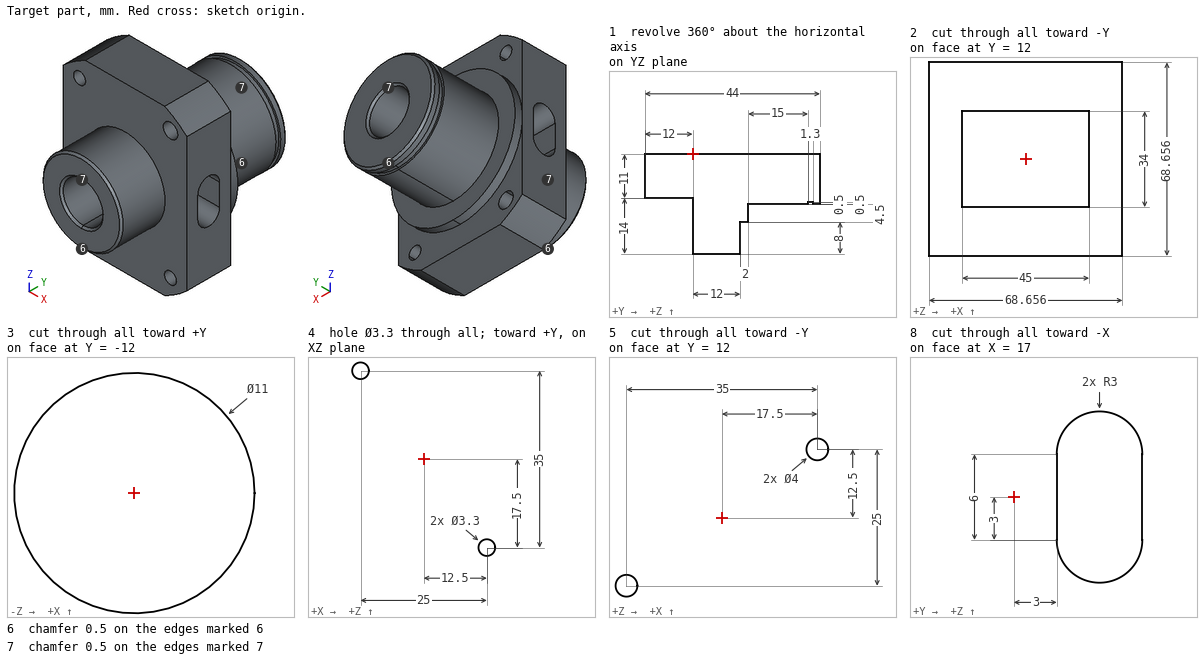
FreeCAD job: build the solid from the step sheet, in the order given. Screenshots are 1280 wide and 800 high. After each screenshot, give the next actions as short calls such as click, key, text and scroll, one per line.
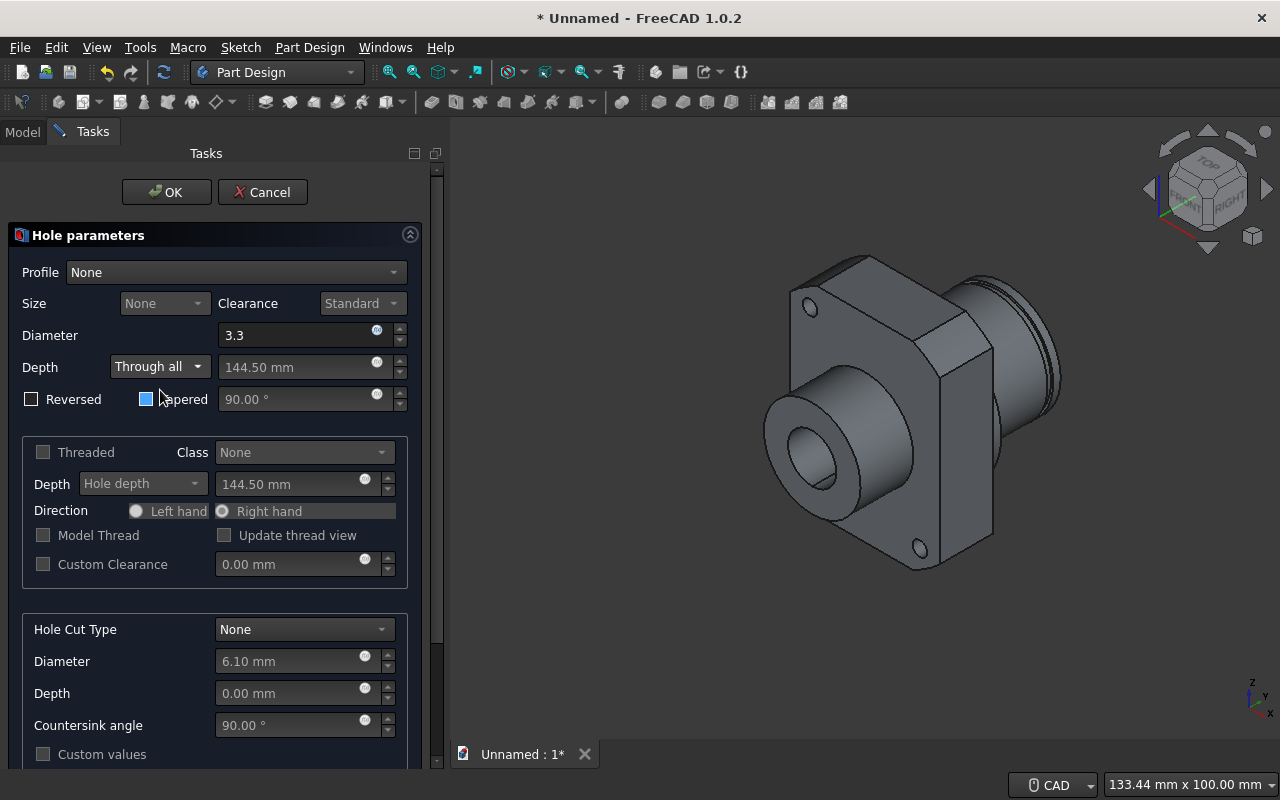
click(167, 192)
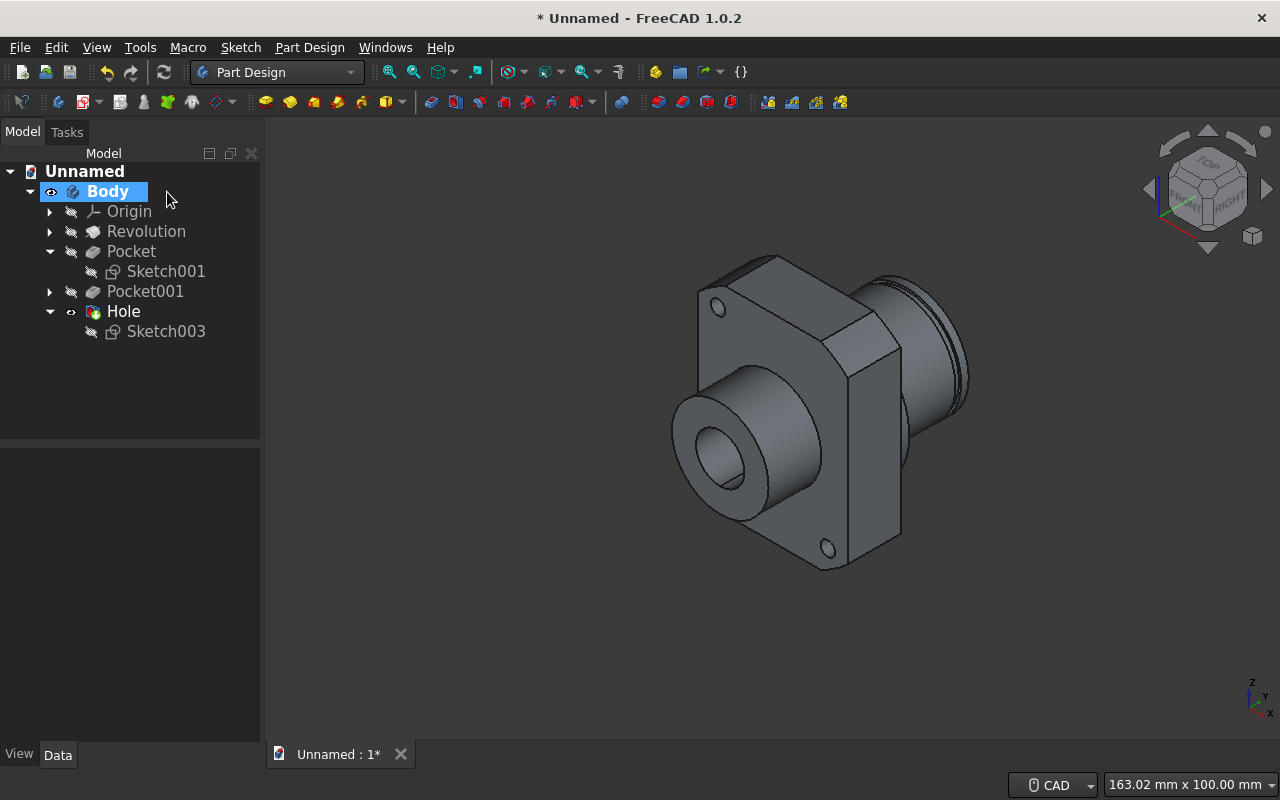
key(4)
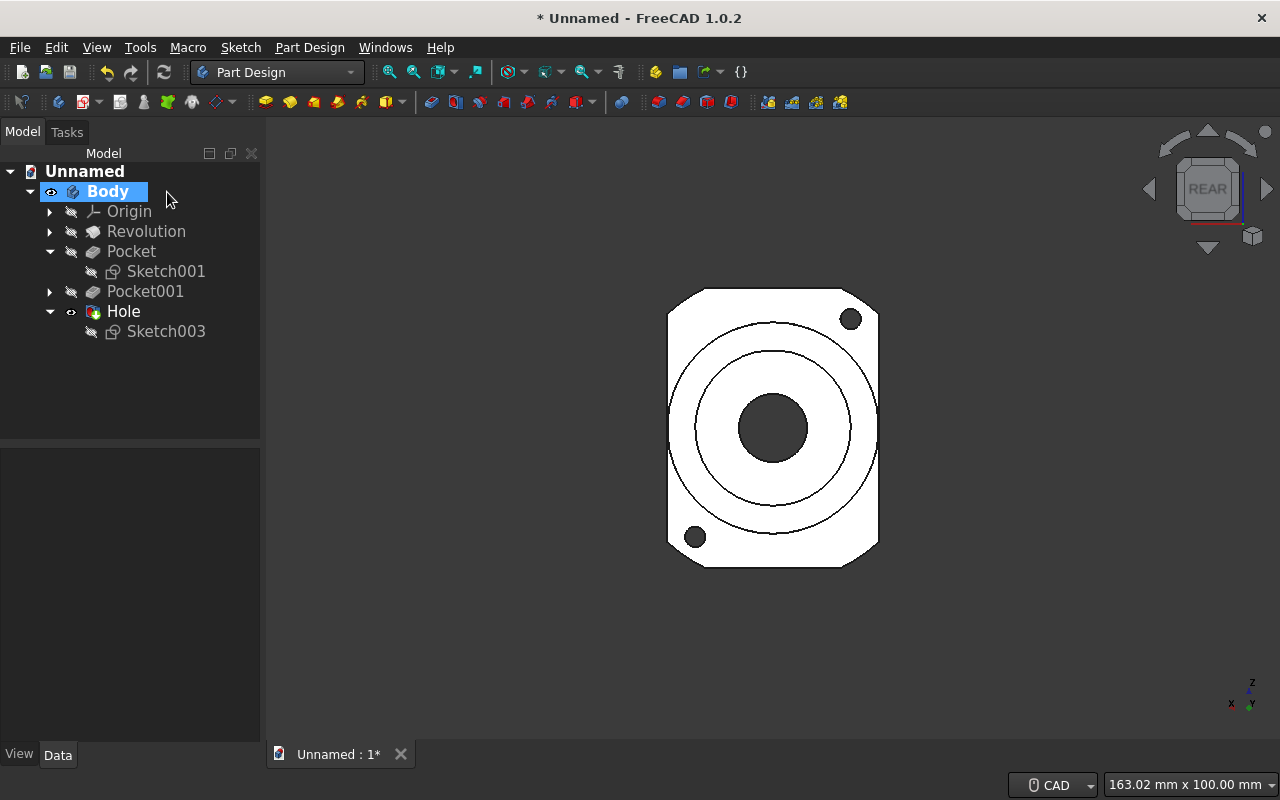
click(713, 317)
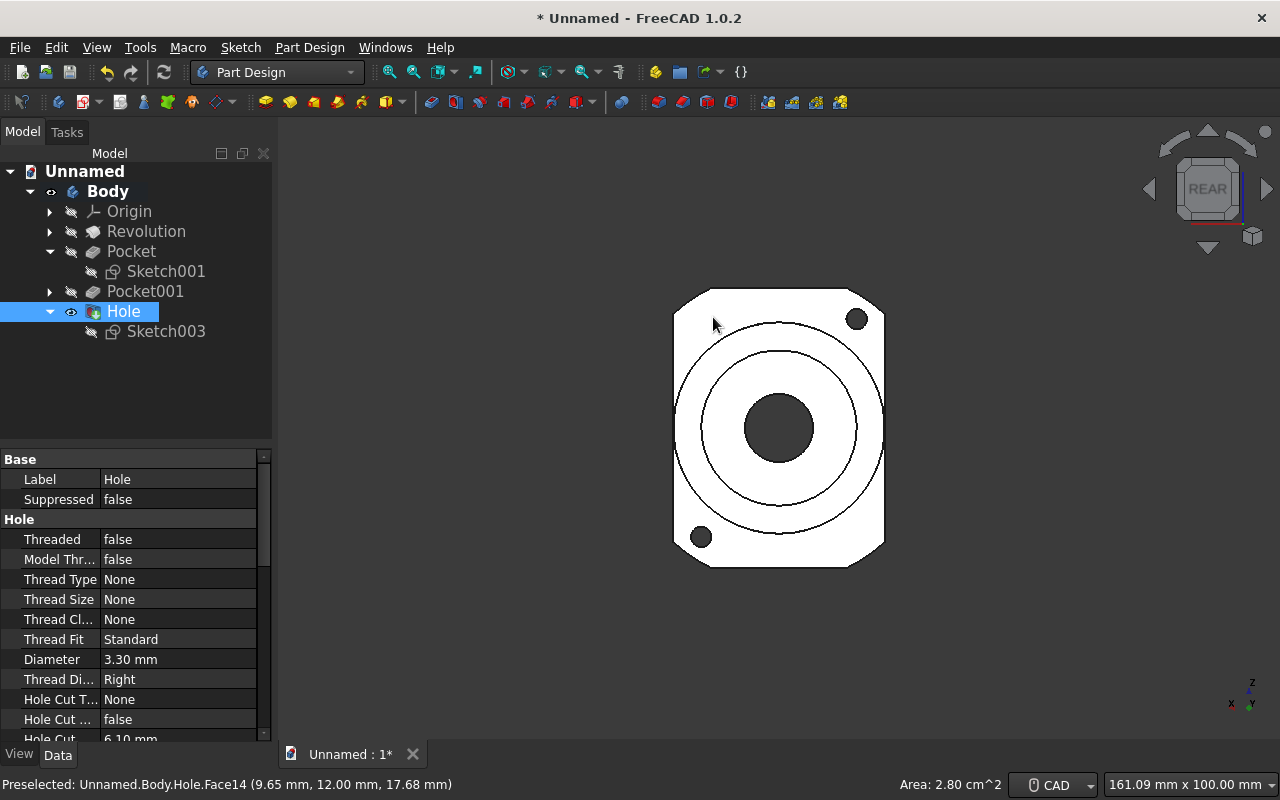
click(84, 102)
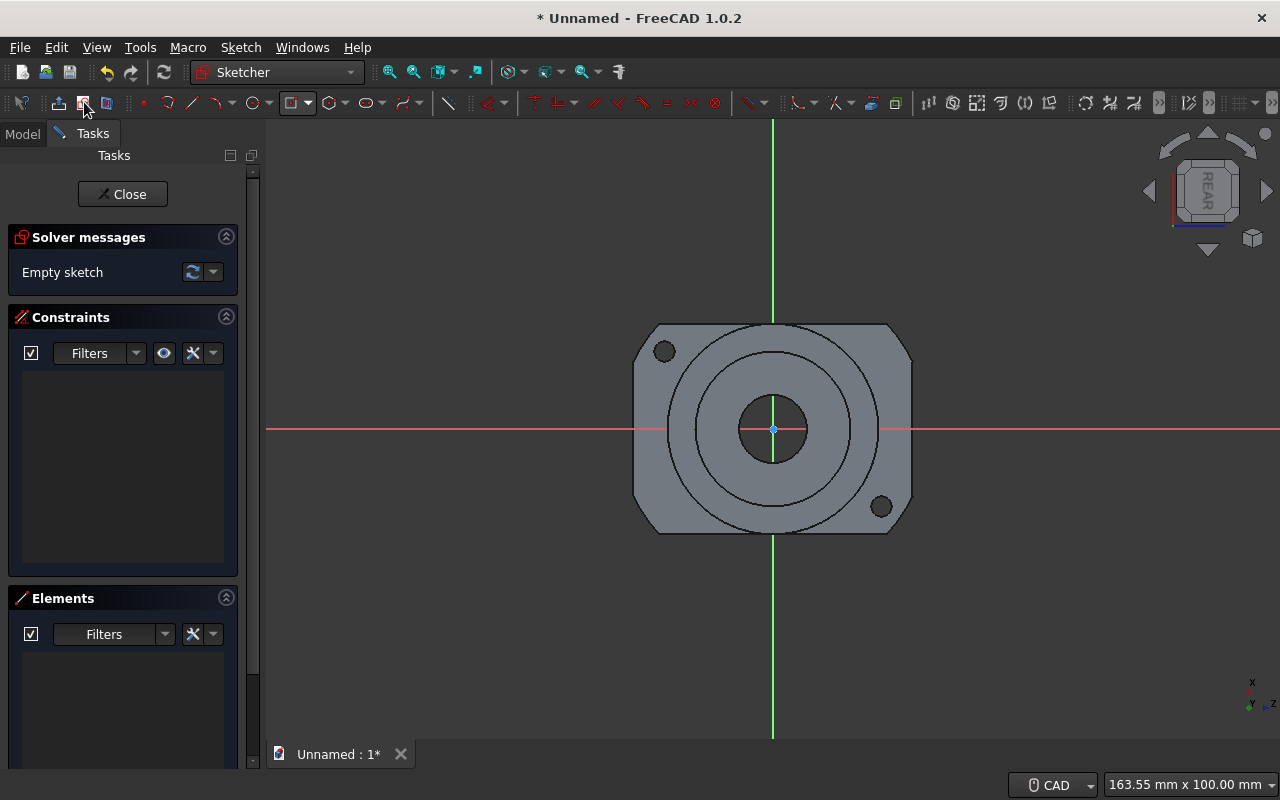
scroll(829, 429, up, 4)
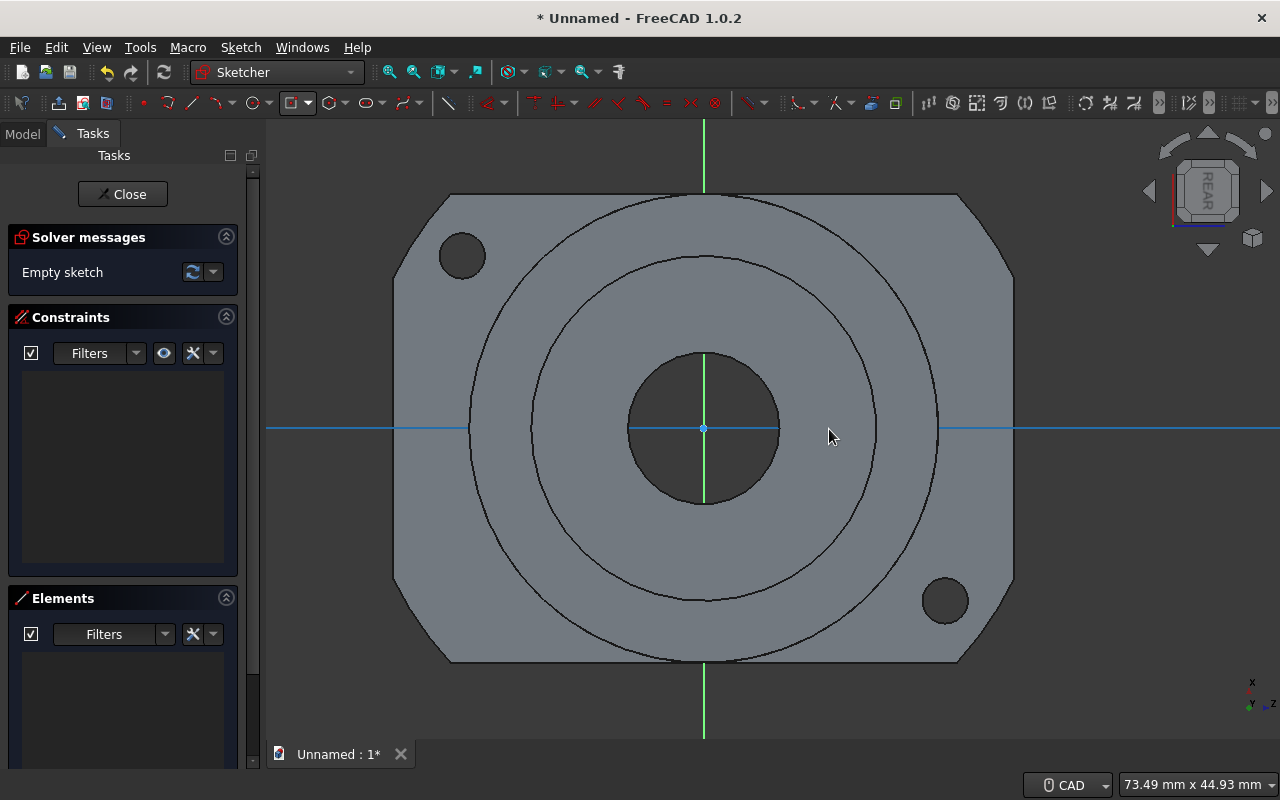
click(254, 104)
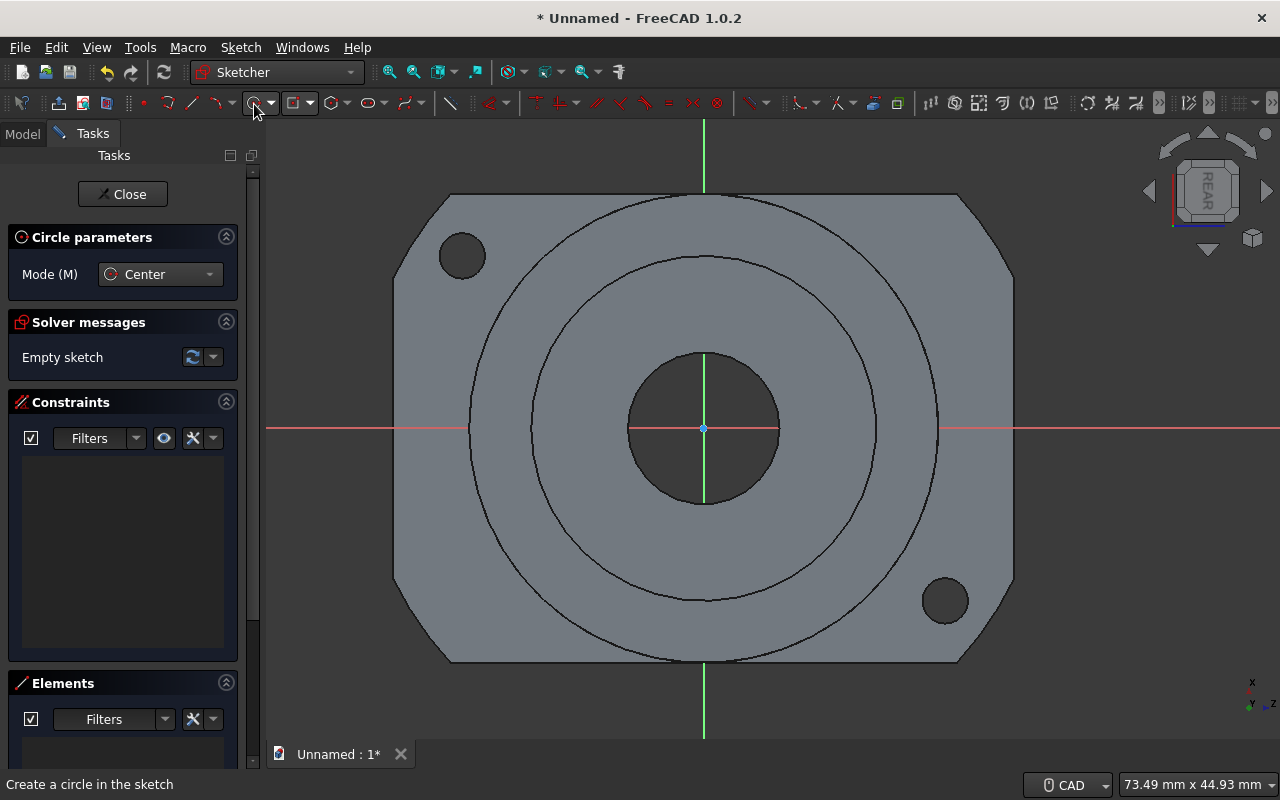
click(945, 256)
move(965, 236)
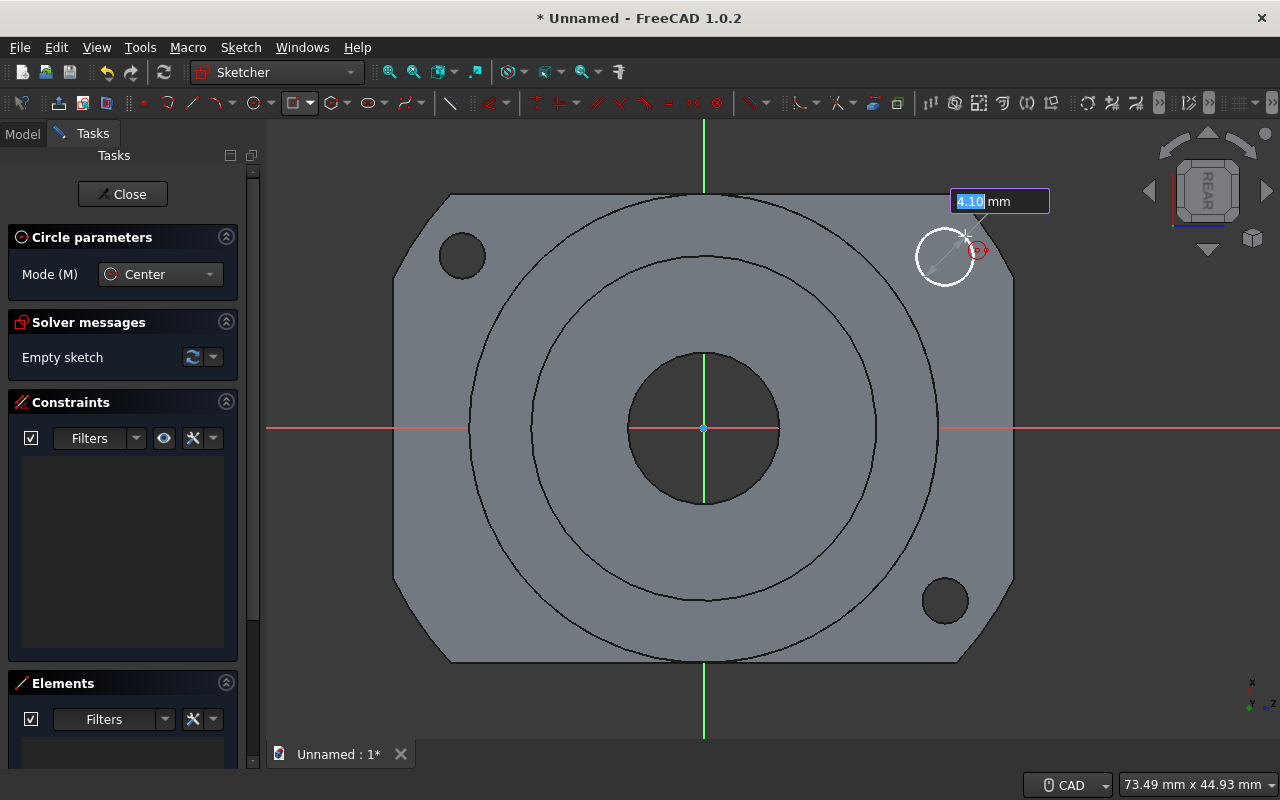
text(4)
key(Return)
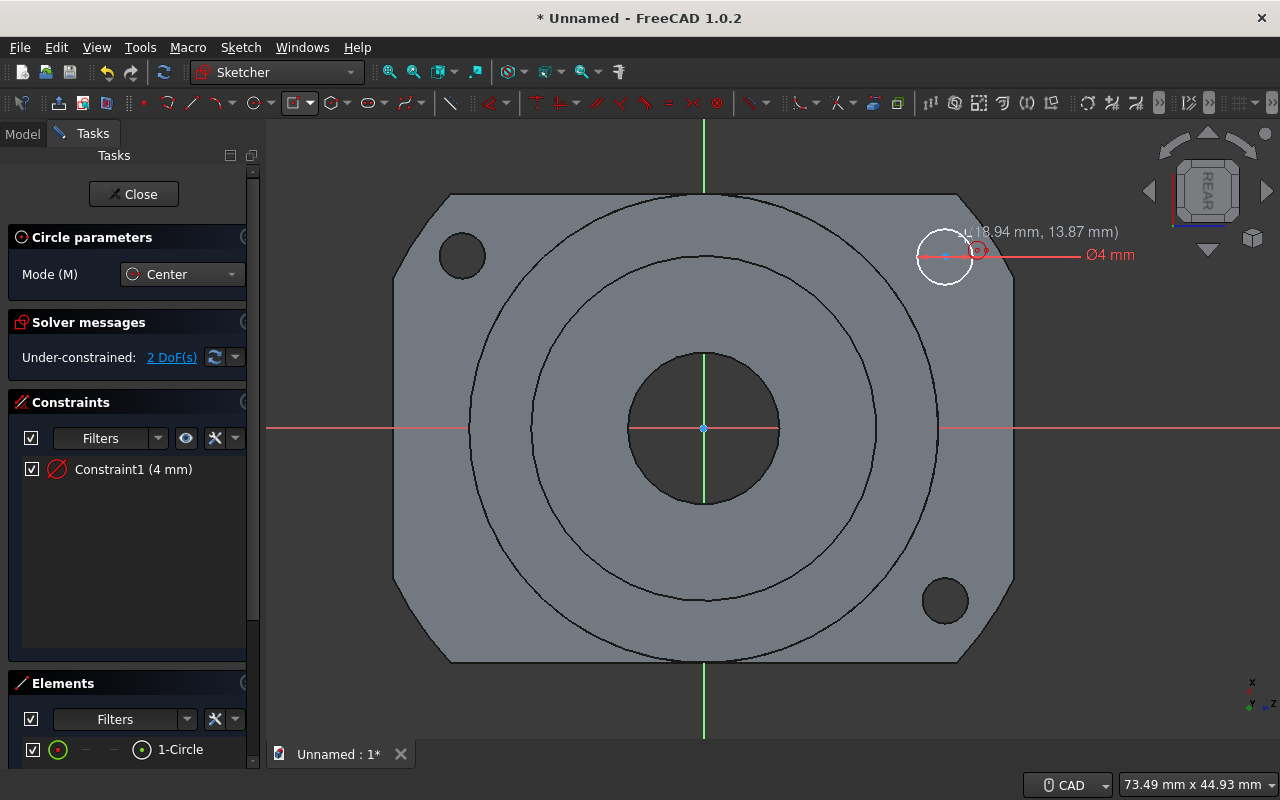
click(462, 601)
move(482, 581)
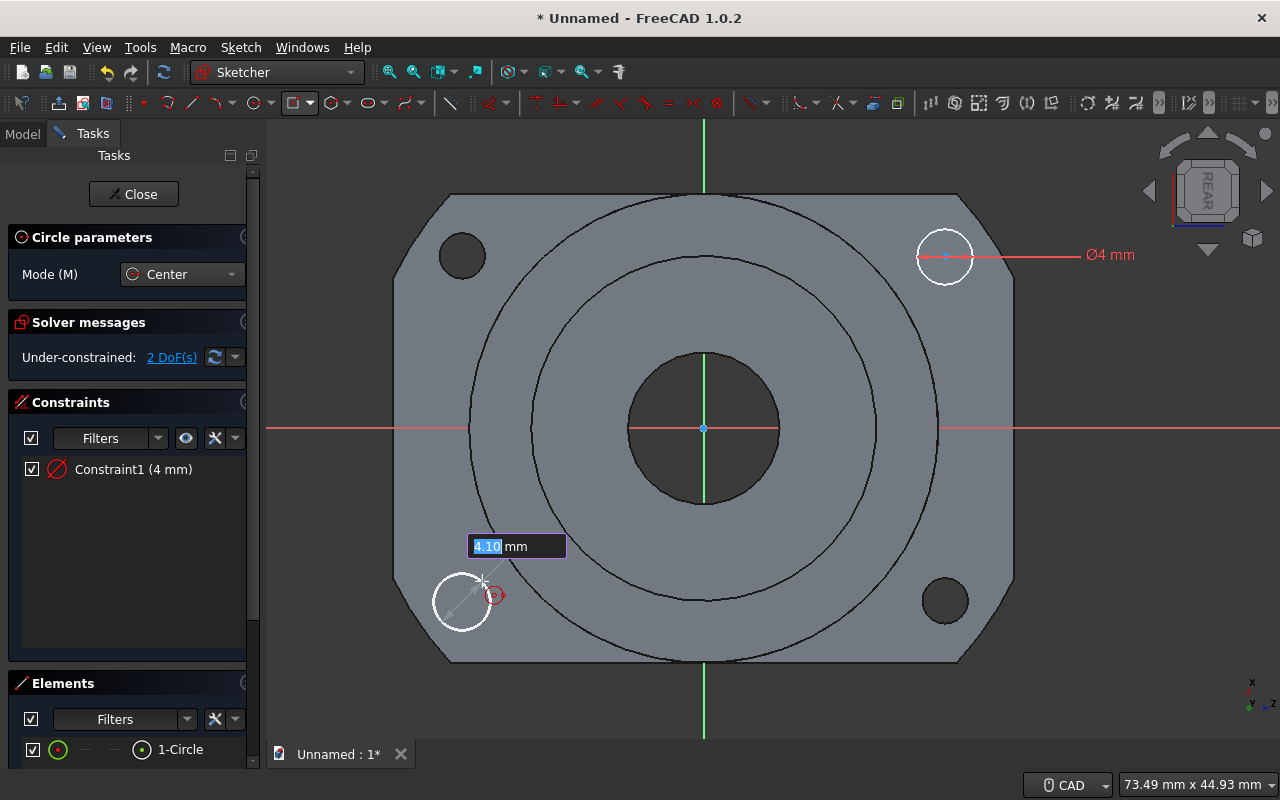
text(4)
key(Return)
key(Escape)